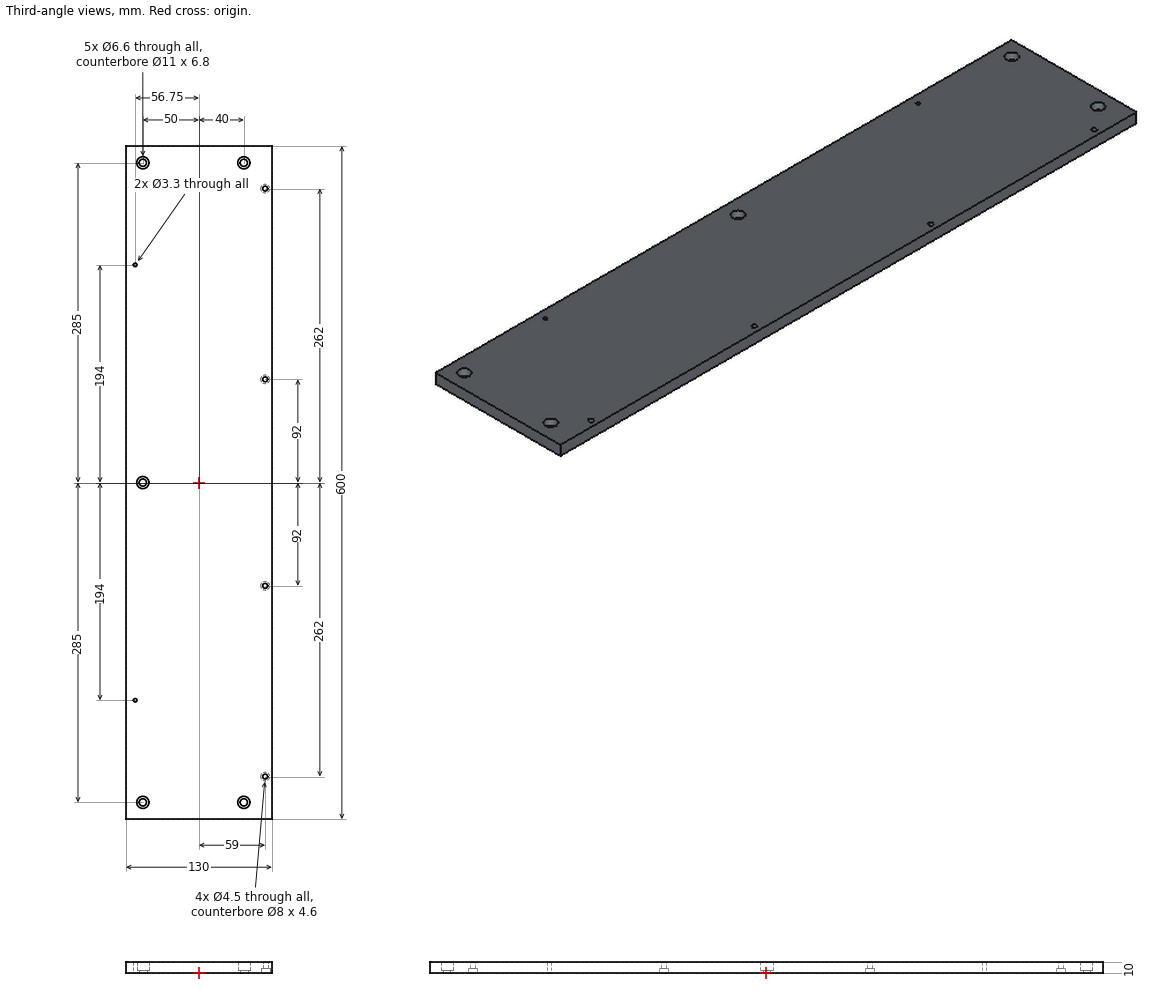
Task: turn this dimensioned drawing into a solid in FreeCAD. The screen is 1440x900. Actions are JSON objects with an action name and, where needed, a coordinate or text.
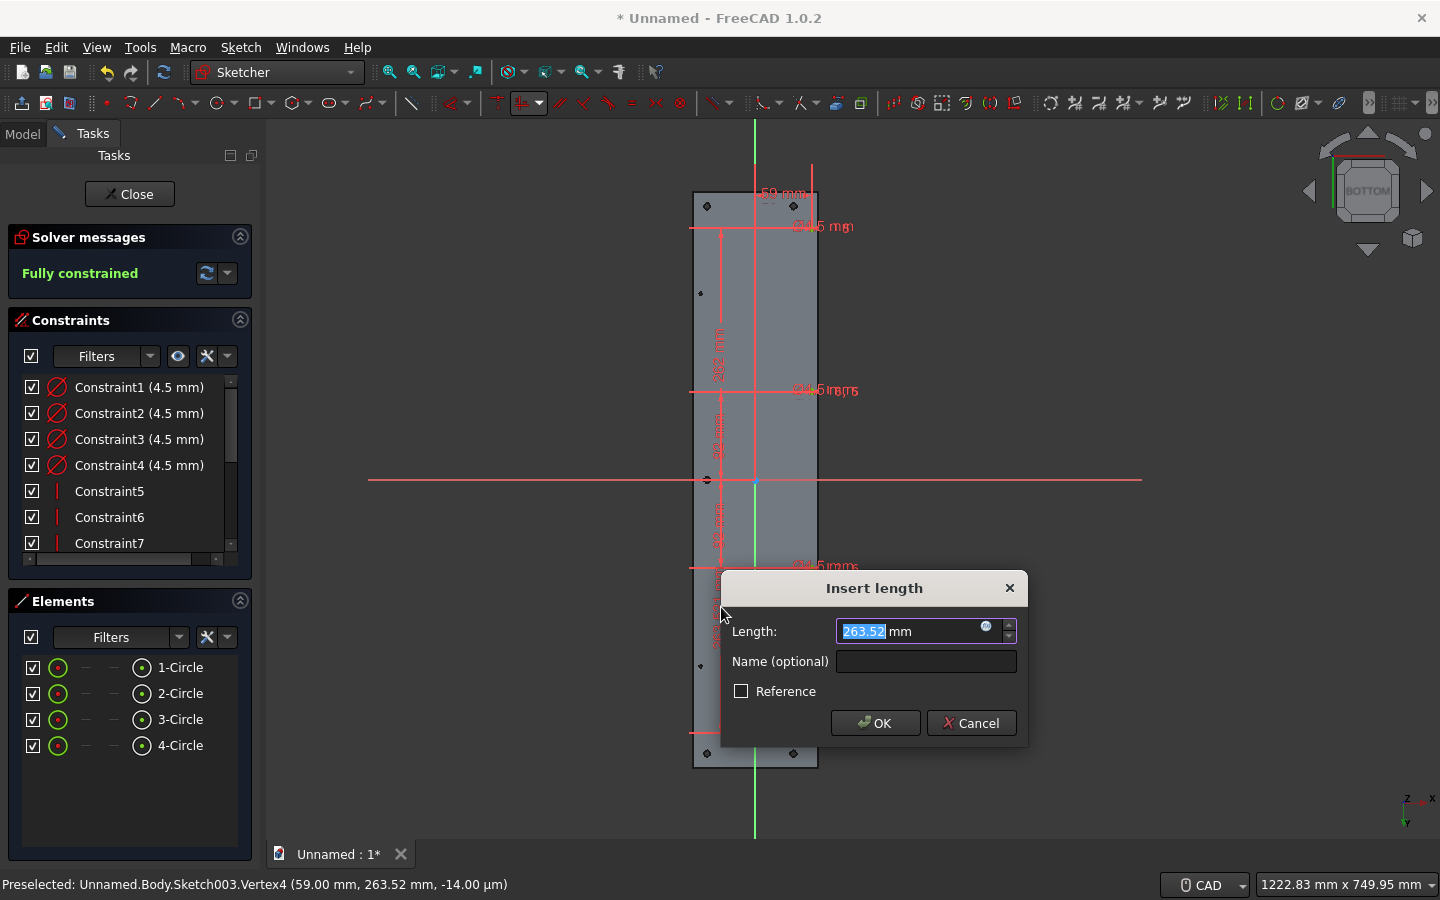
{"action": "type", "text": "262"}
{"action": "key", "text": "Return"}
{"action": "key", "text": "Escape"}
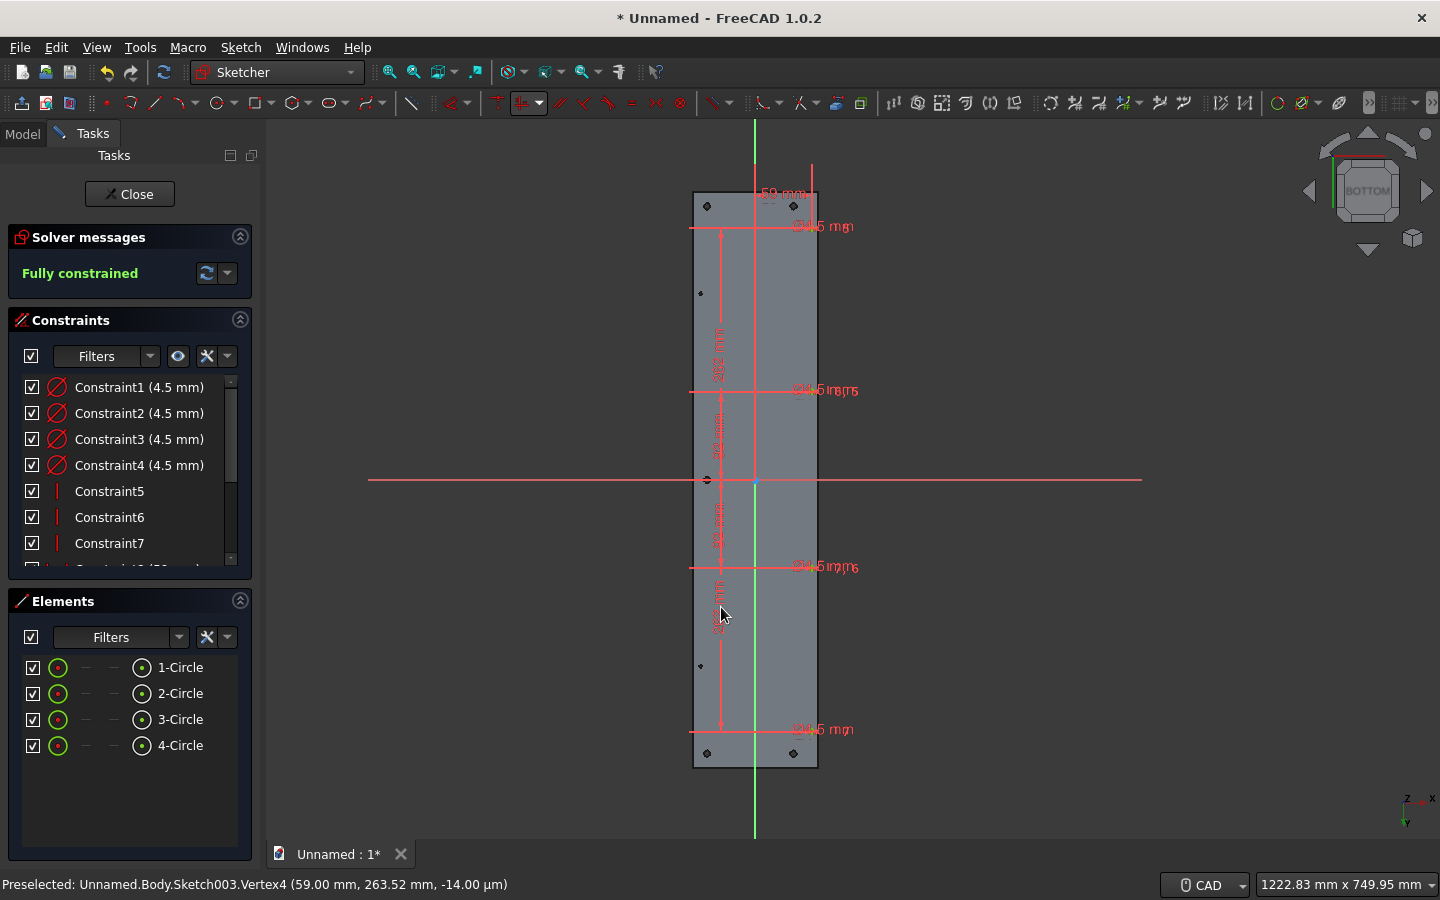
{"action": "left_click", "coordinate": [130, 194]}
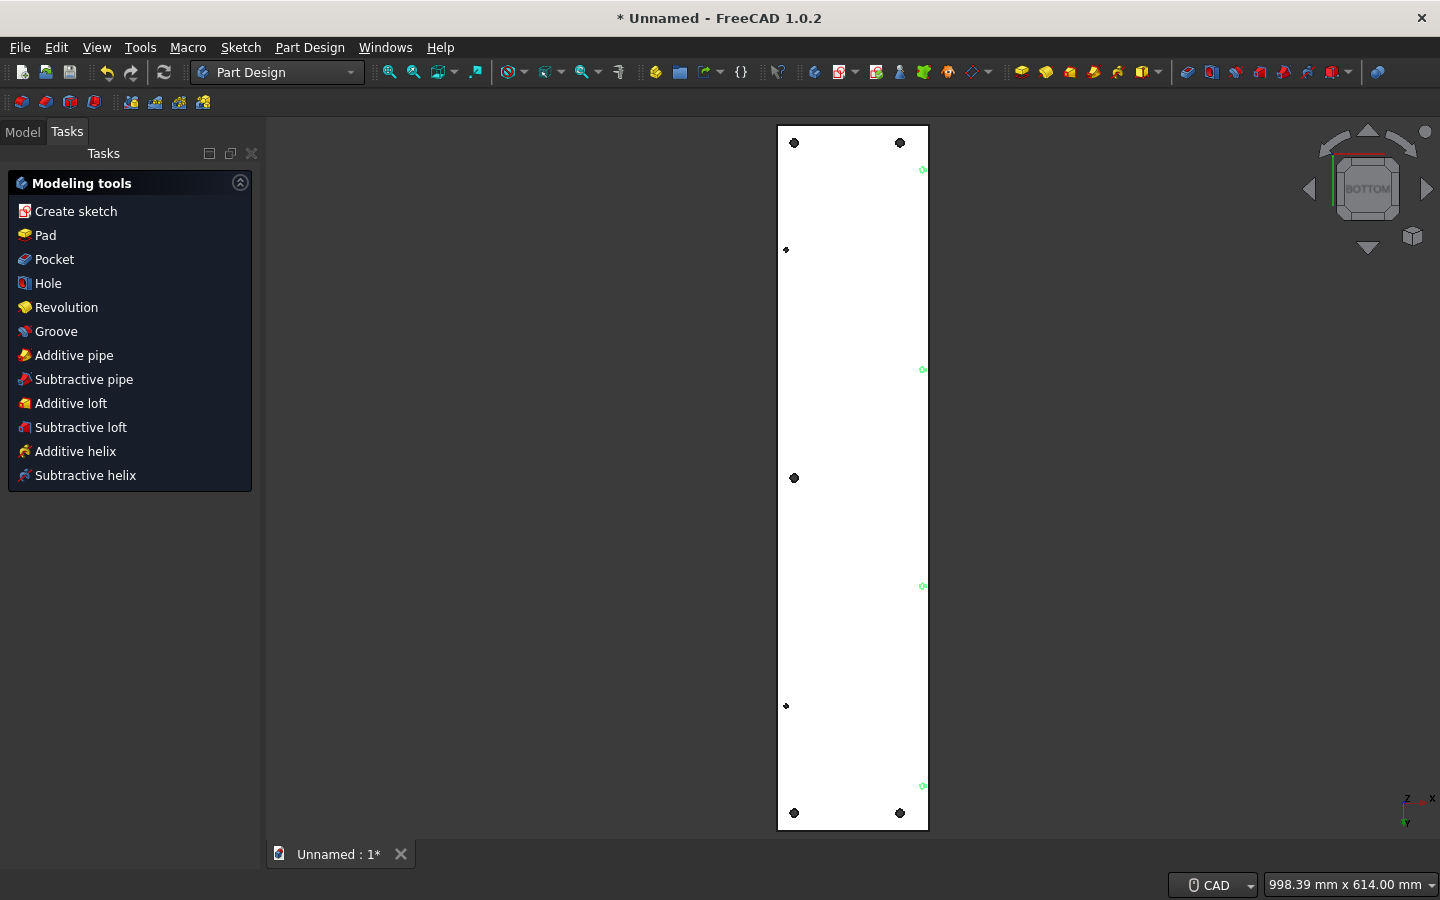
{"action": "left_click", "coordinate": [1212, 72]}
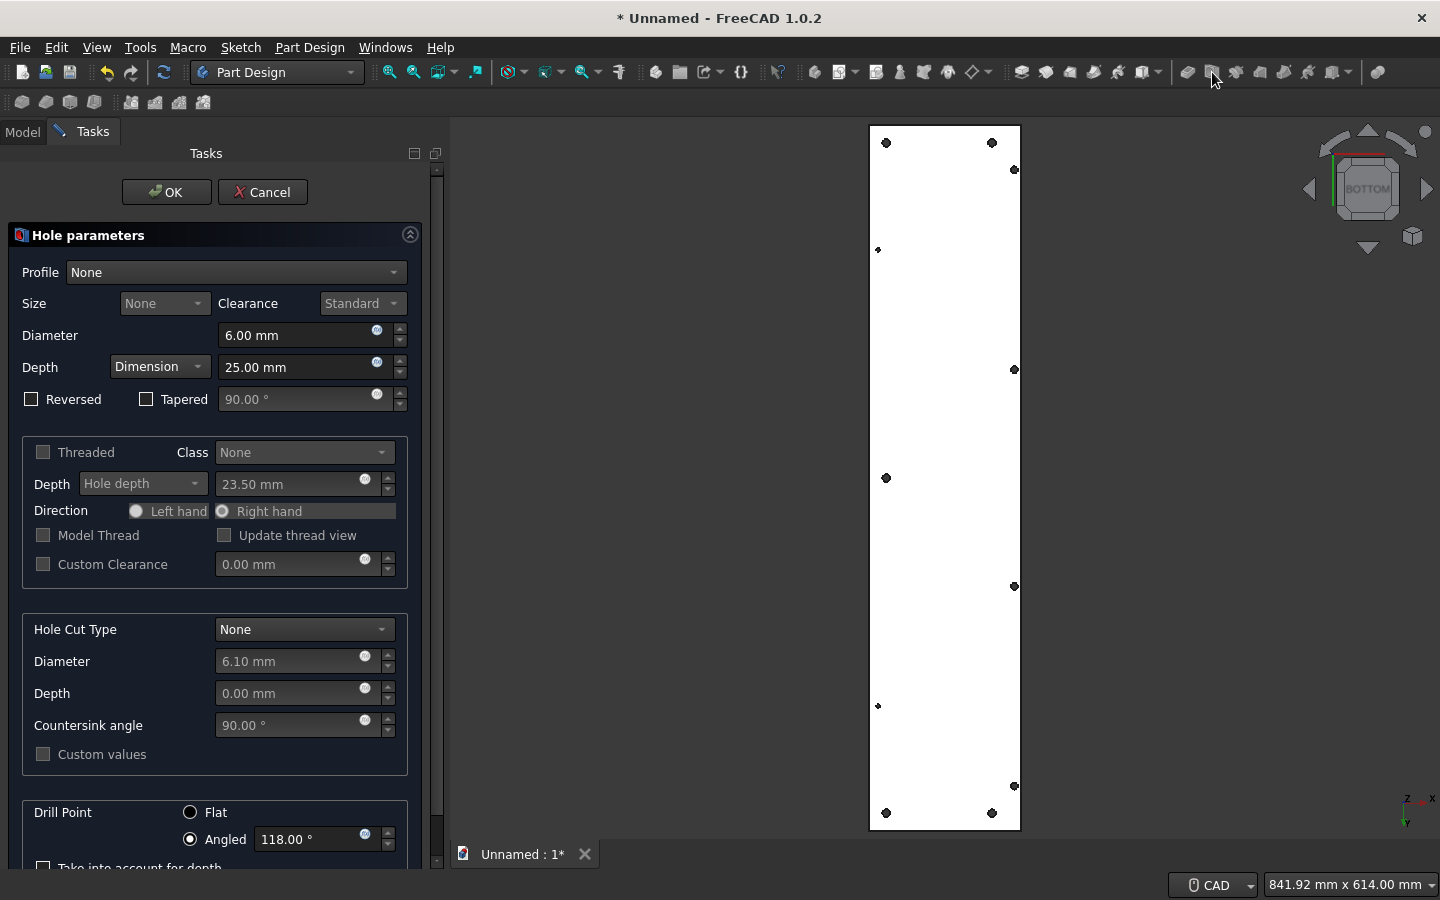
{"action": "triple_click", "coordinate": [305, 335]}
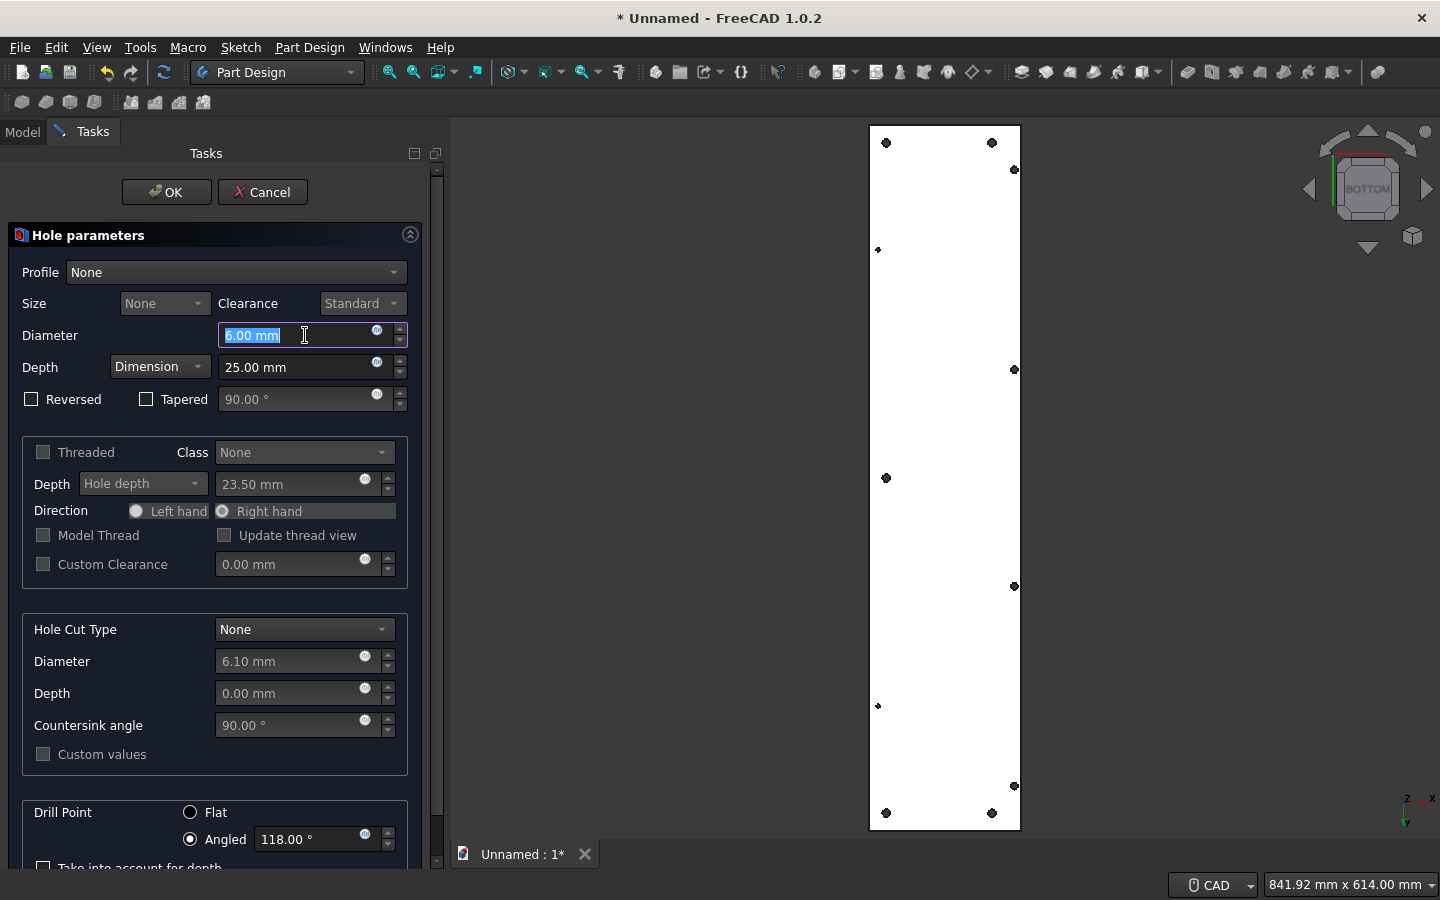
{"action": "type", "text": "4.5"}
{"action": "key", "text": "Tab"}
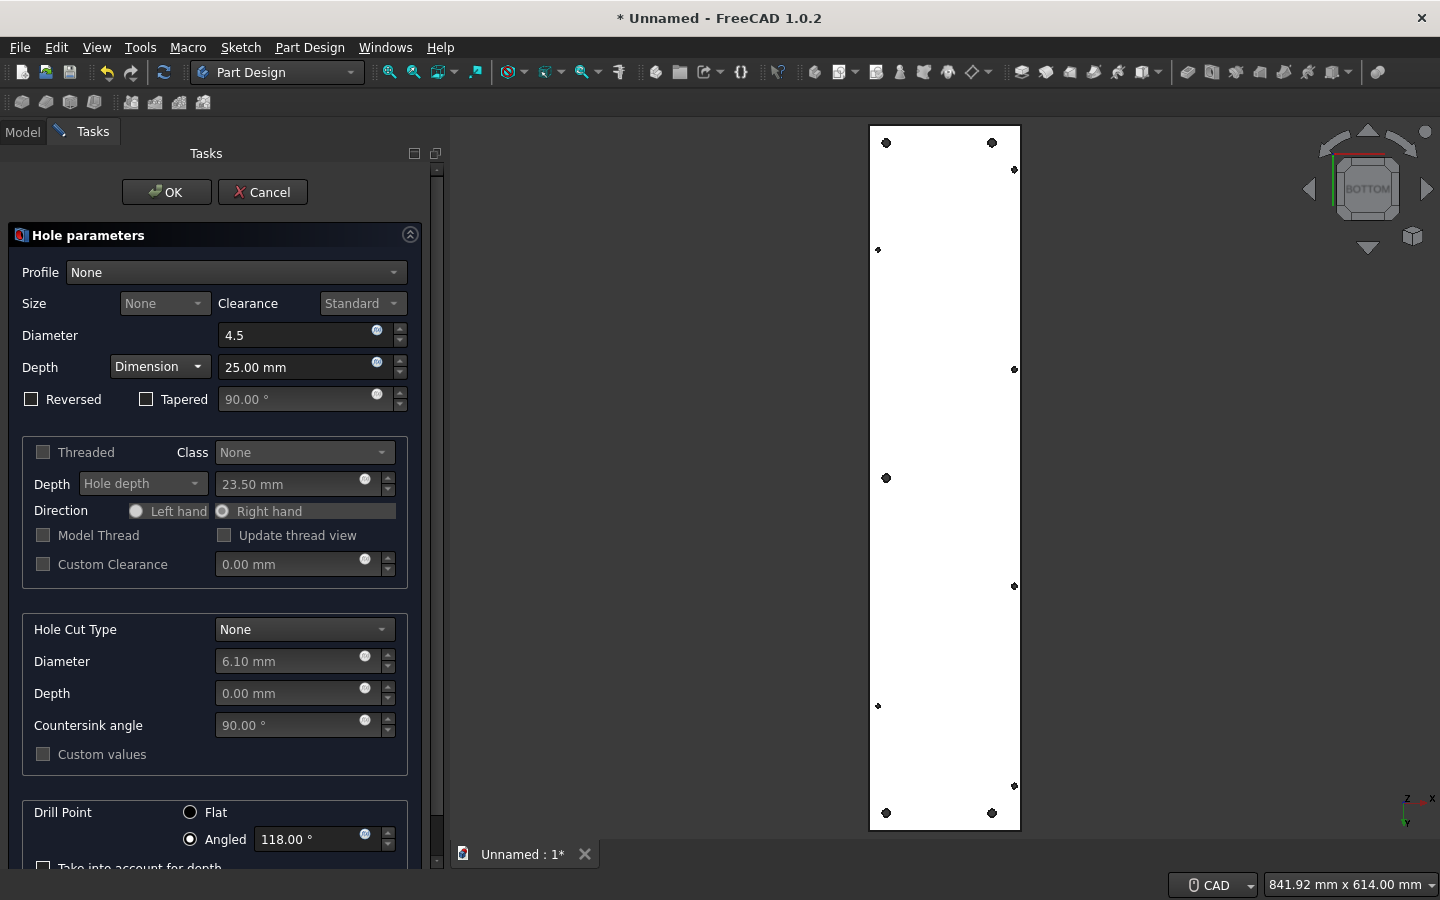
{"action": "left_click", "coordinate": [161, 366]}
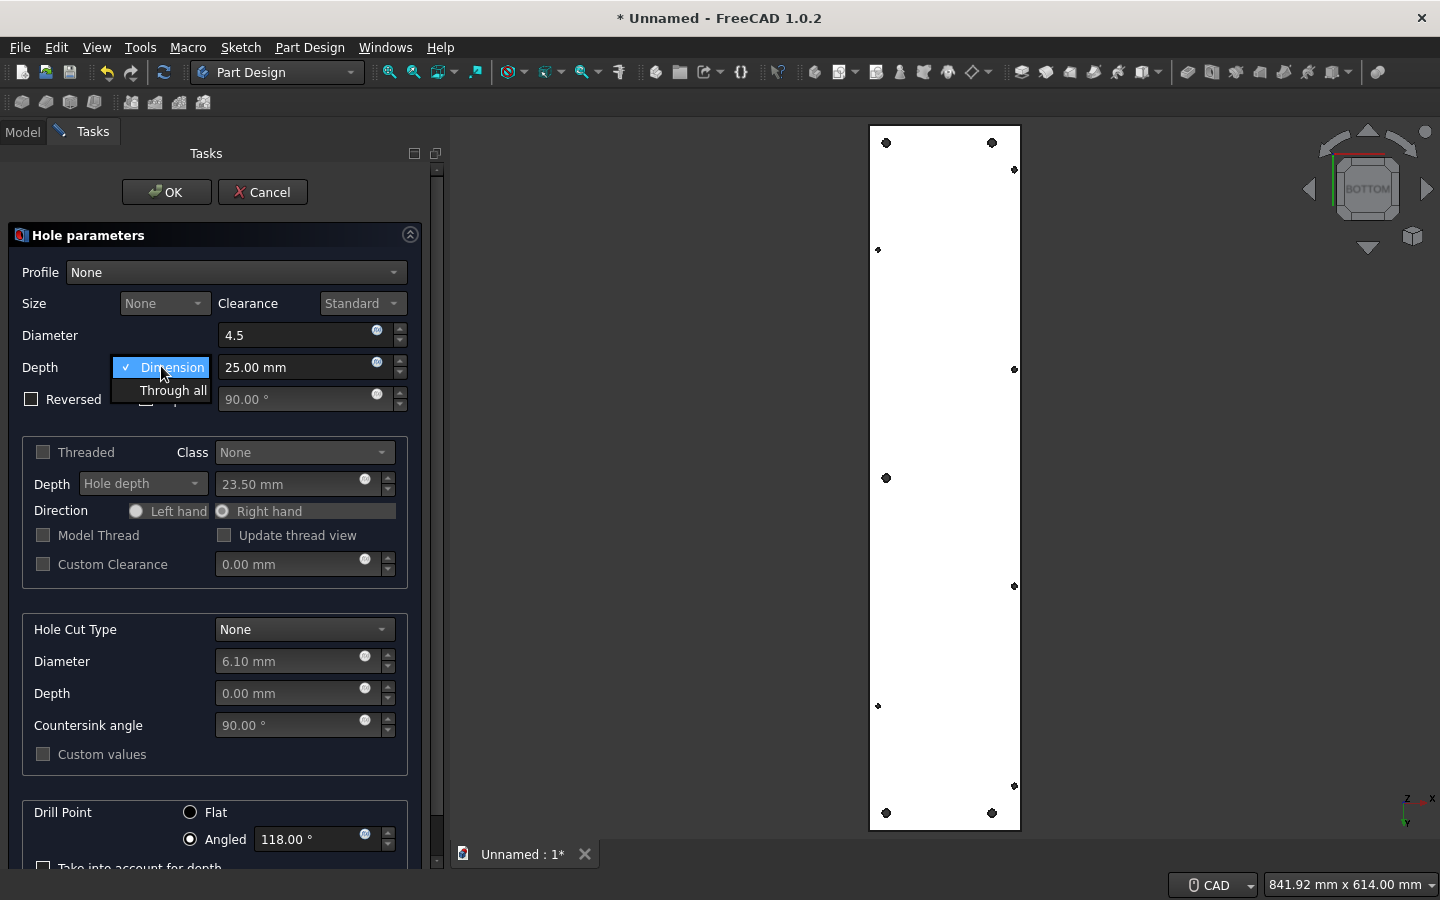
{"action": "left_click", "coordinate": [160, 390]}